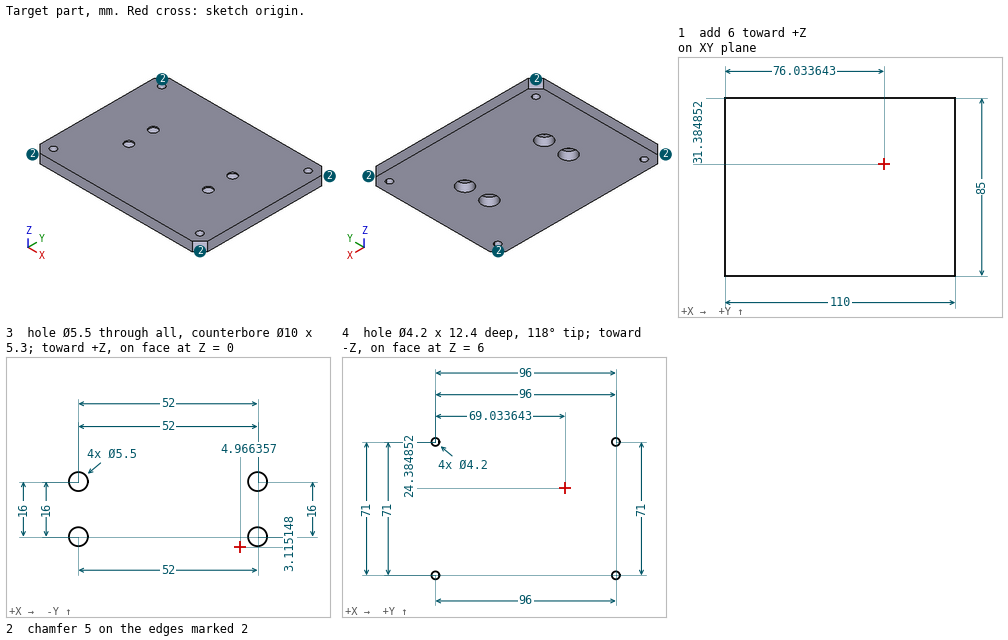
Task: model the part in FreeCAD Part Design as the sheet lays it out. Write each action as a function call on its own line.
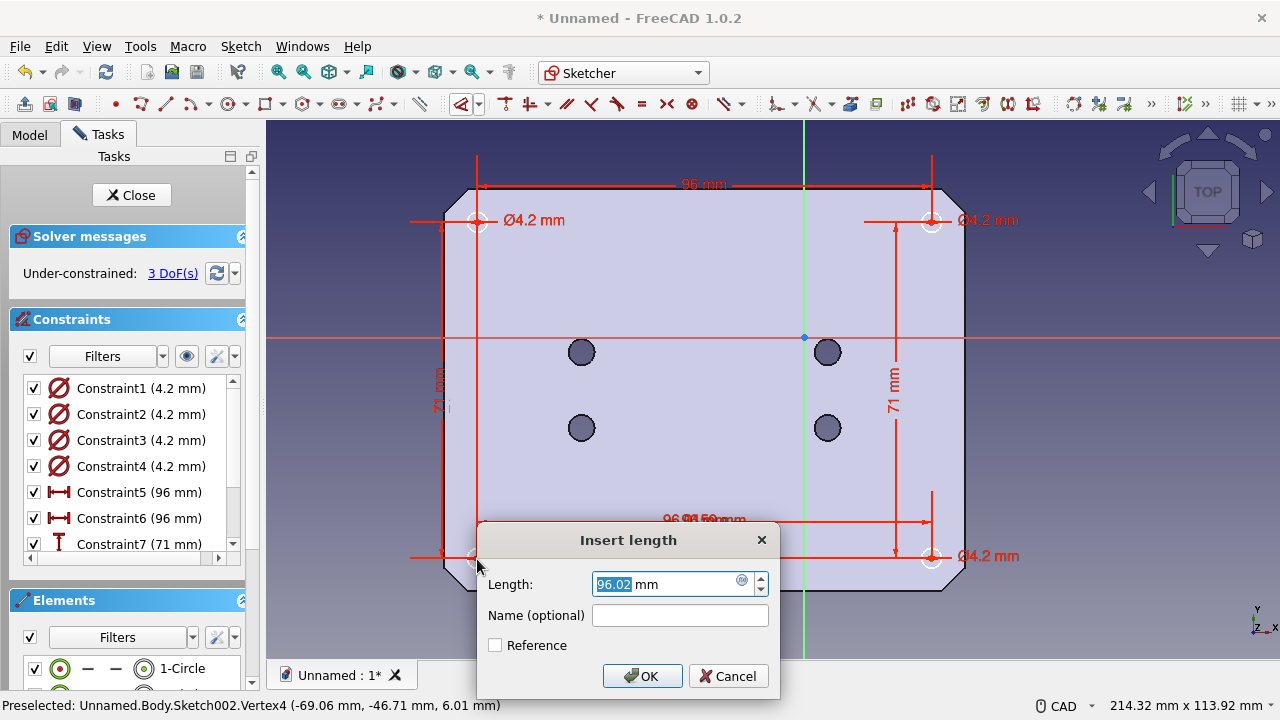
text(96)
key(Return)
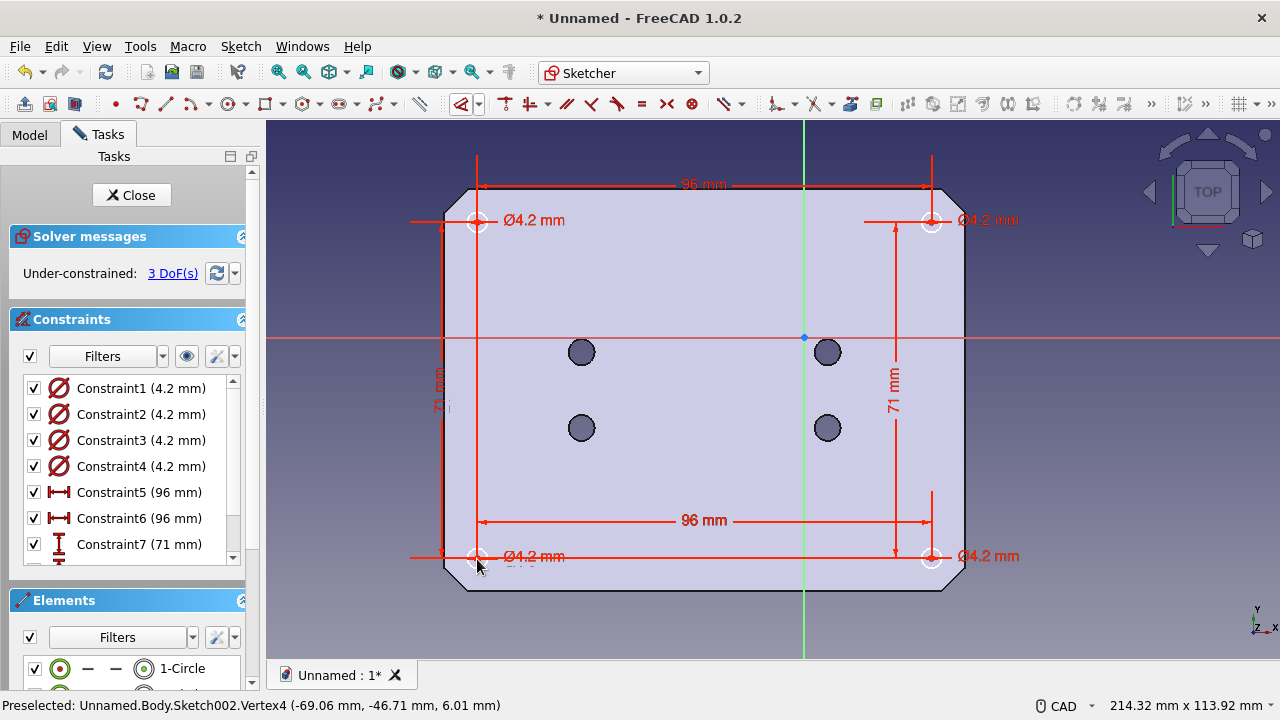
click(477, 222)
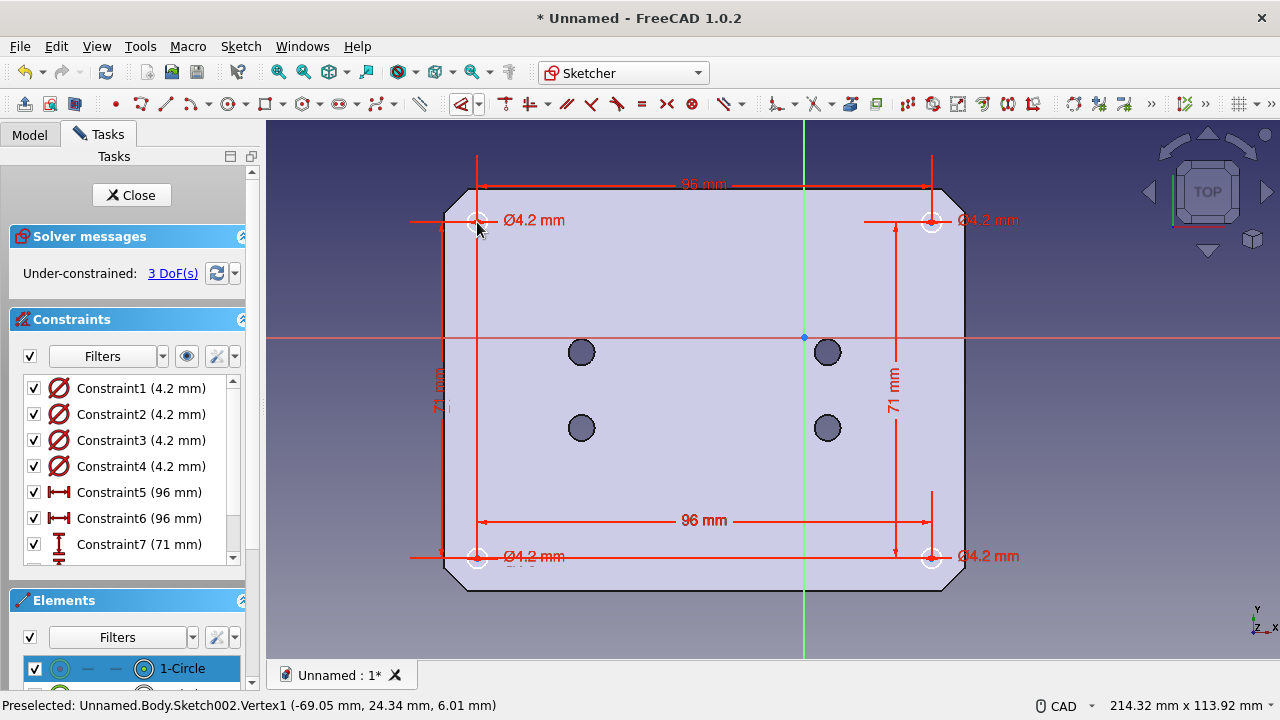
click(477, 559)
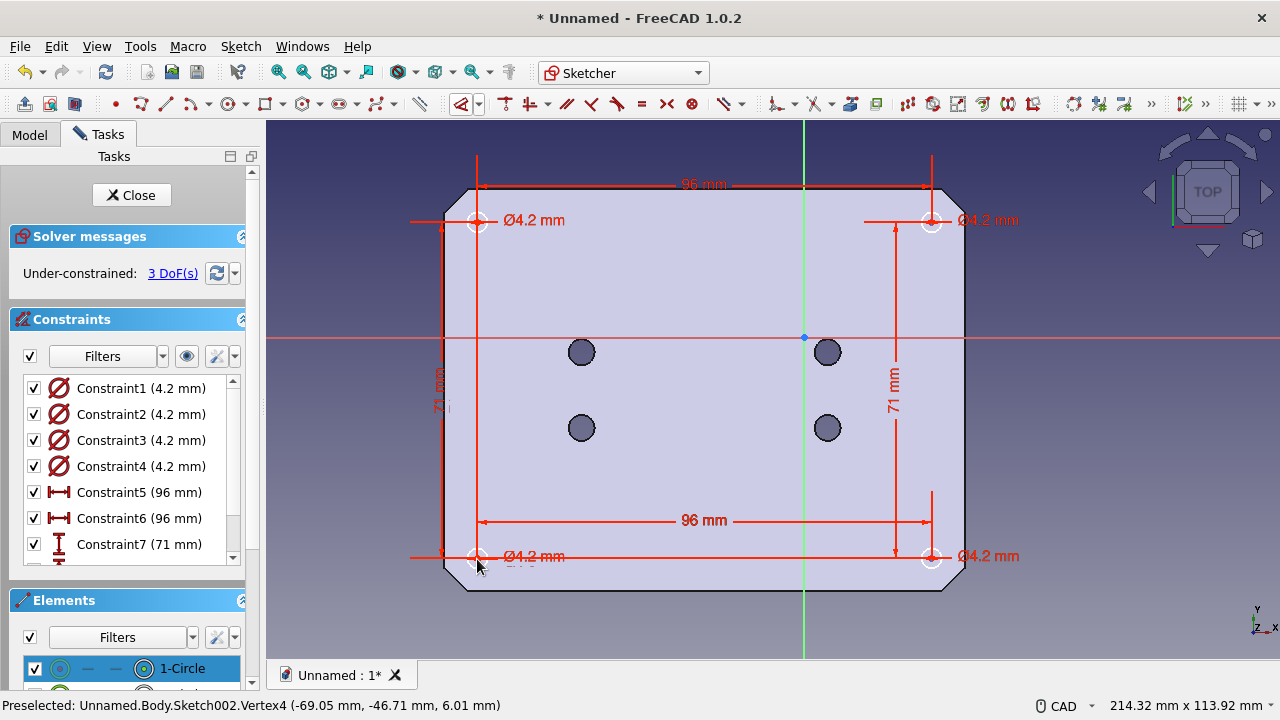
click(478, 104)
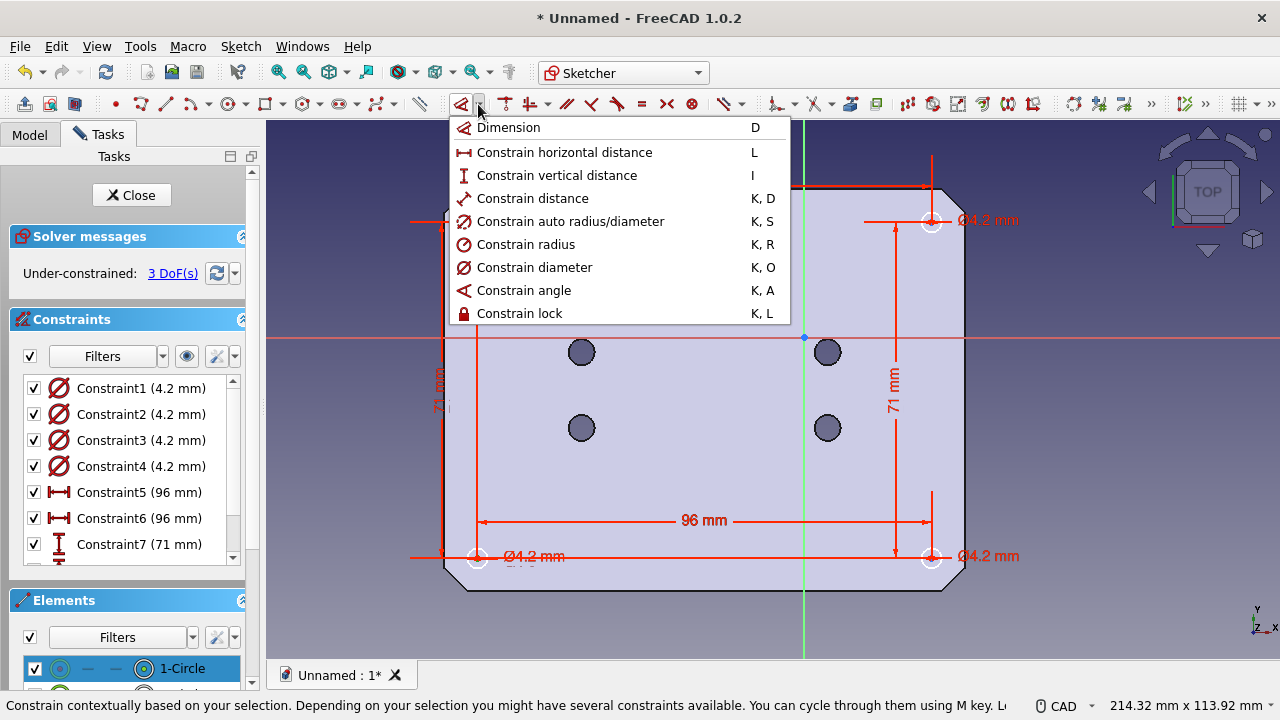
click(620, 176)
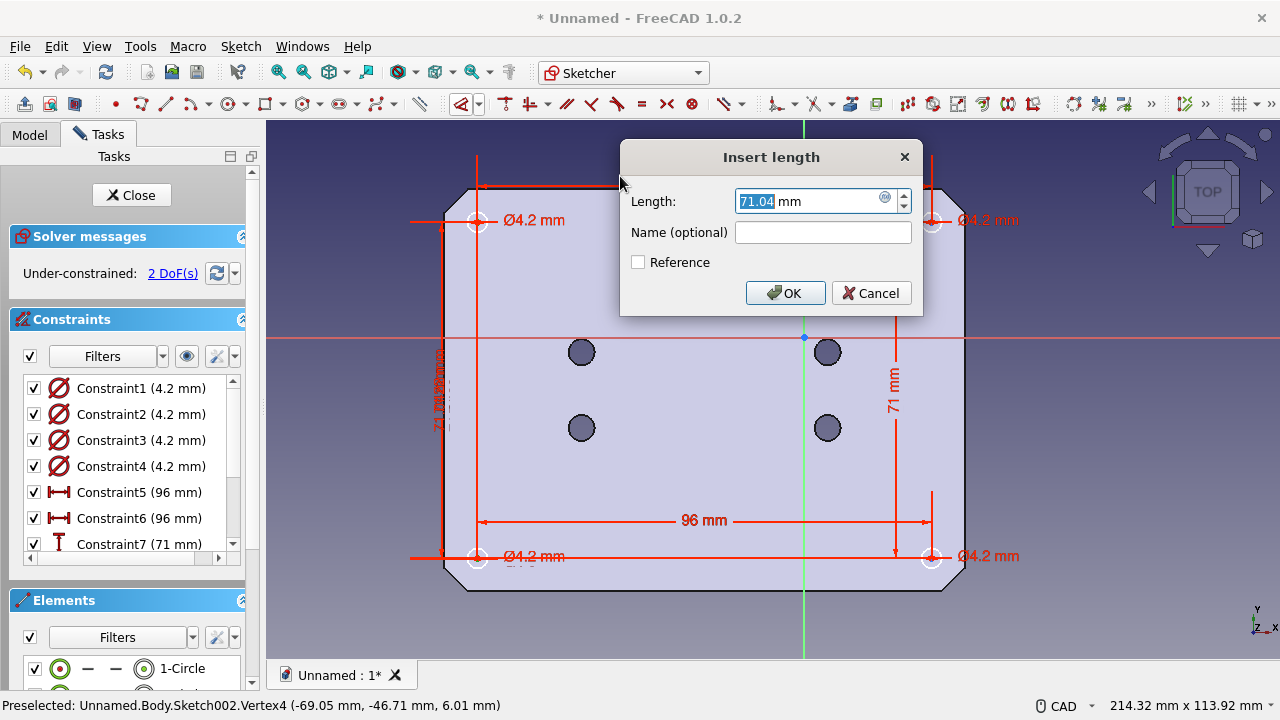
text(71)
key(Return)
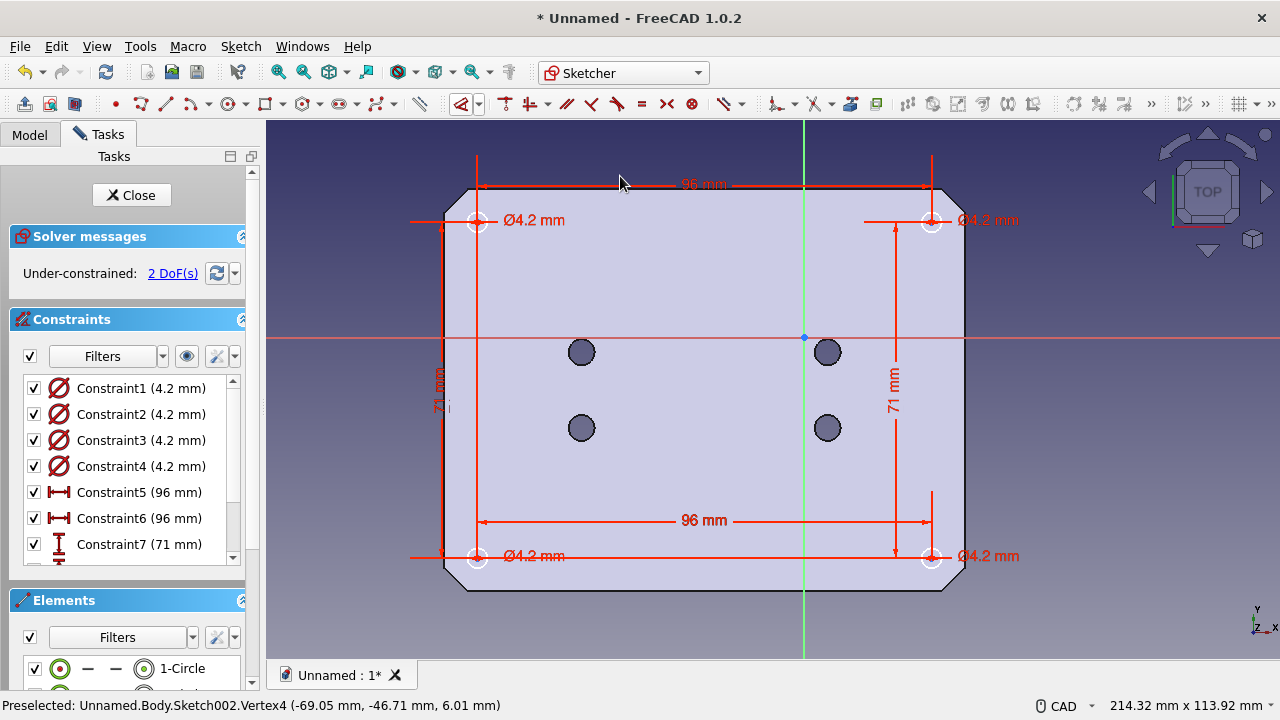
click(477, 222)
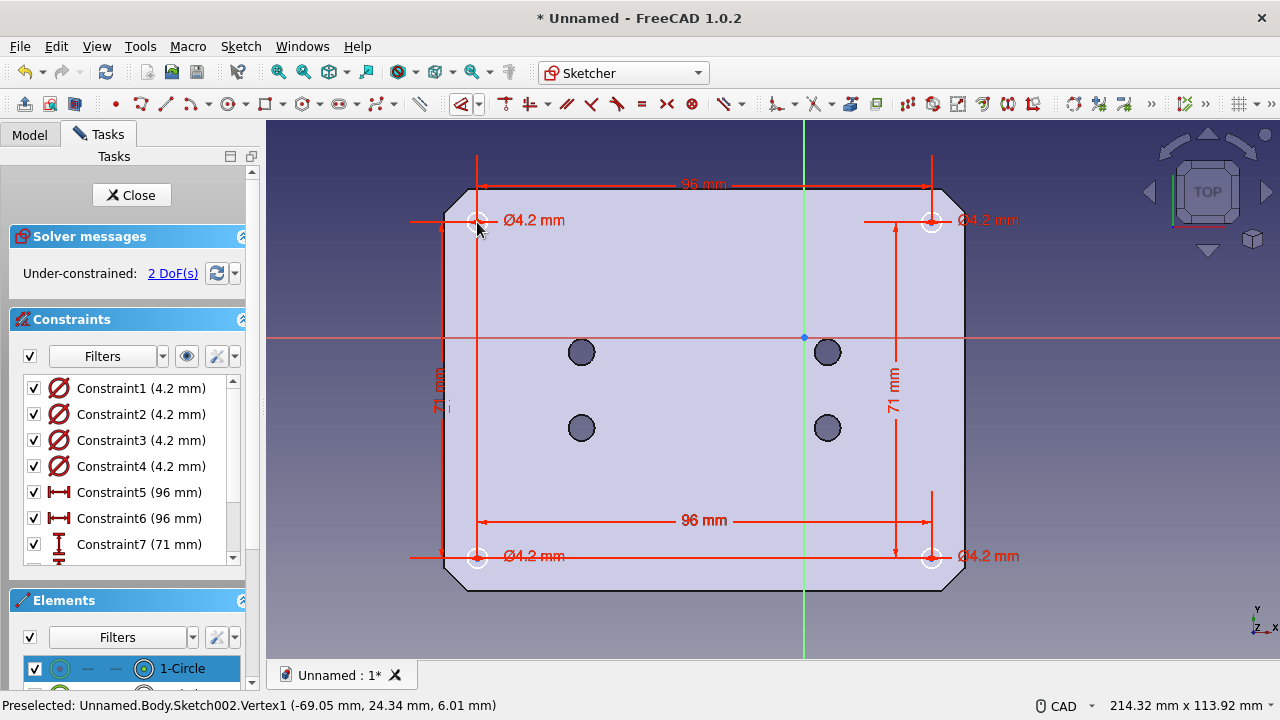
key(l)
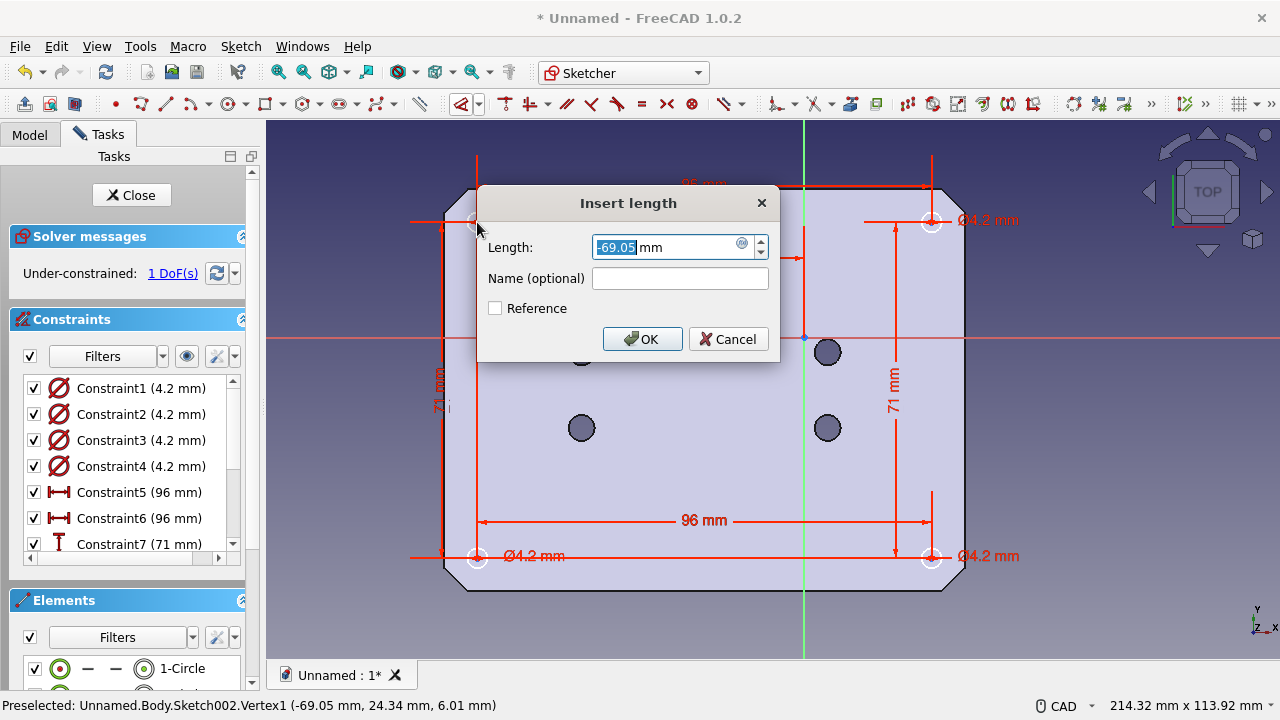
text(-69.033643)
key(Return)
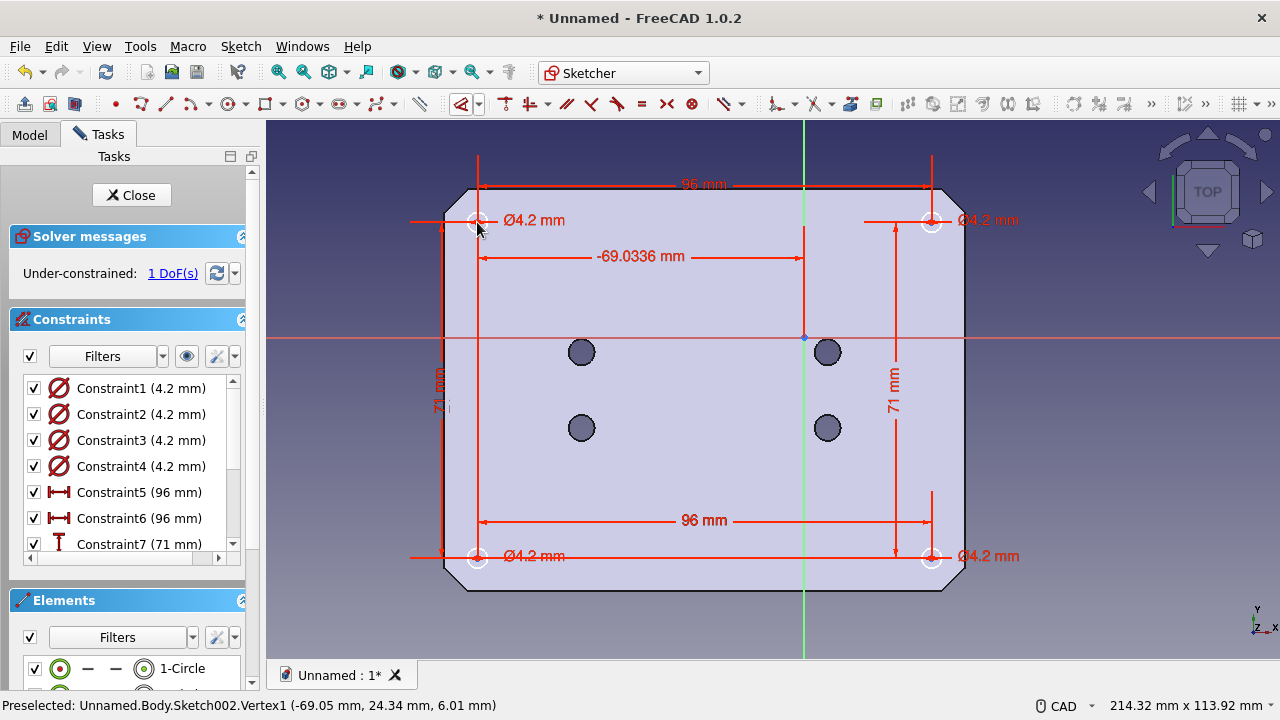
click(478, 222)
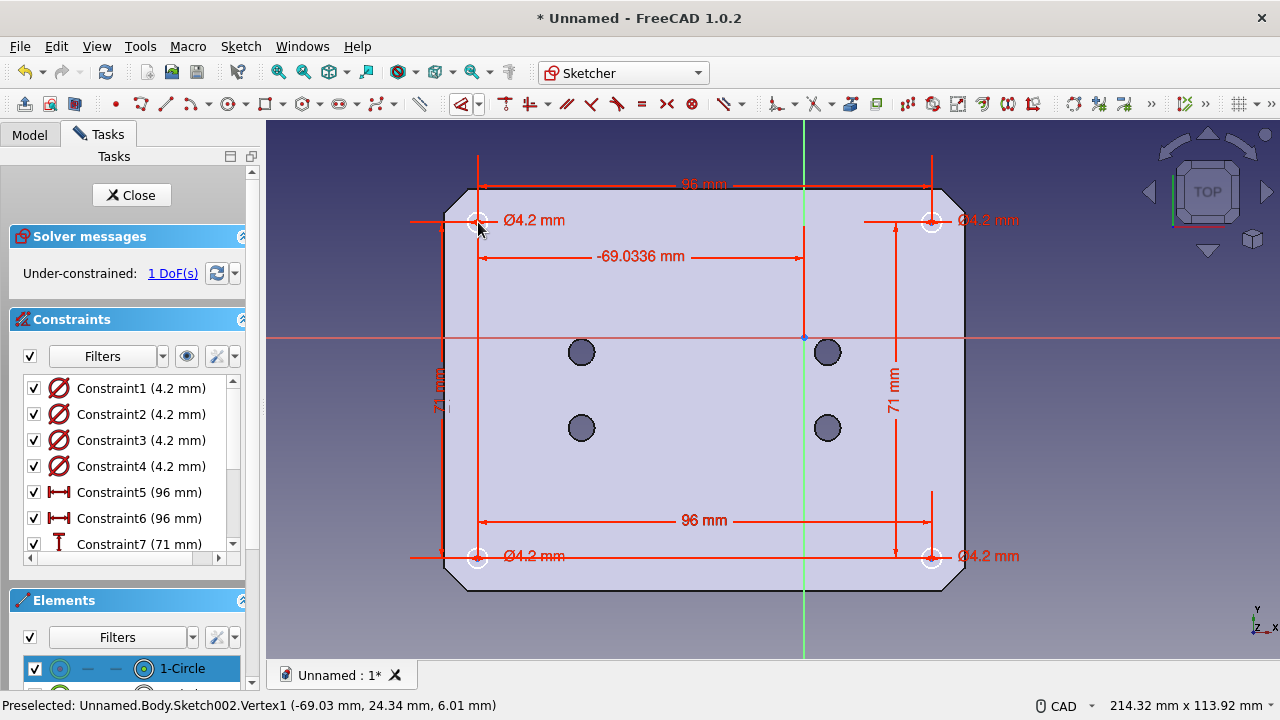
click(478, 104)